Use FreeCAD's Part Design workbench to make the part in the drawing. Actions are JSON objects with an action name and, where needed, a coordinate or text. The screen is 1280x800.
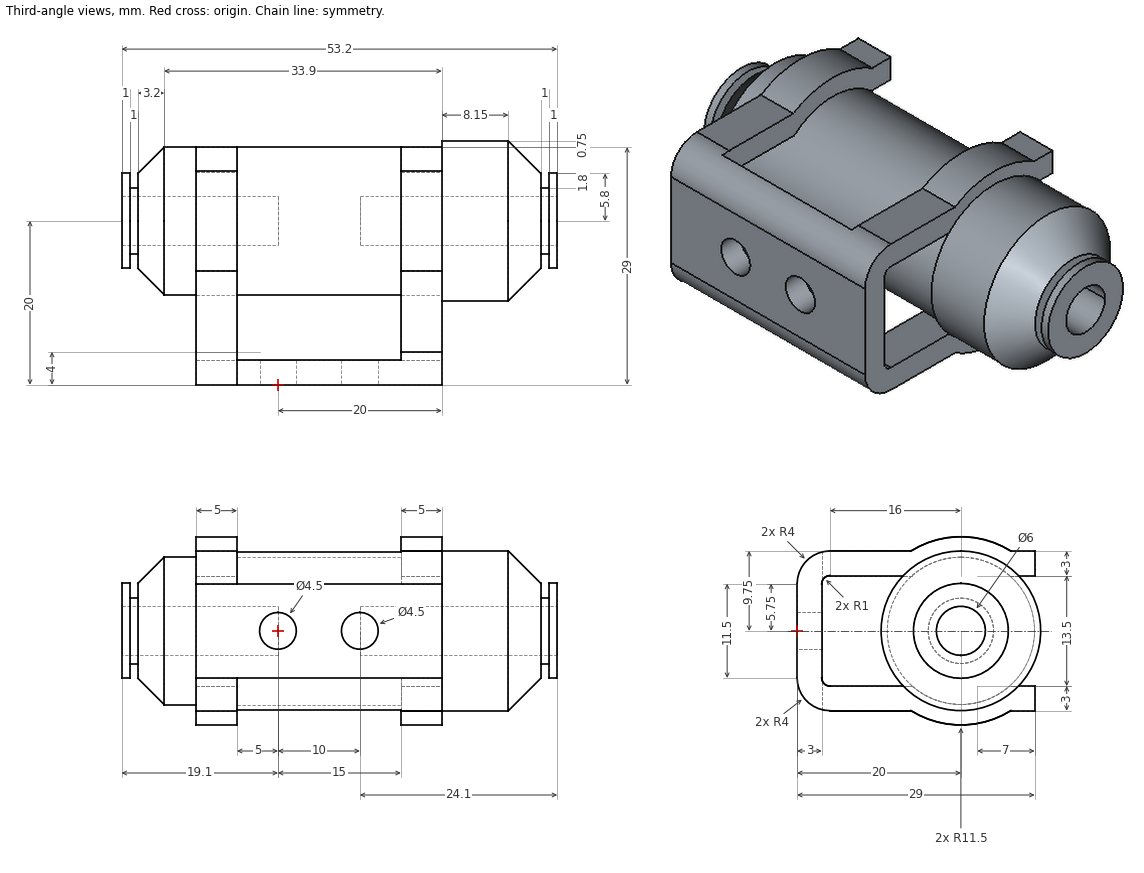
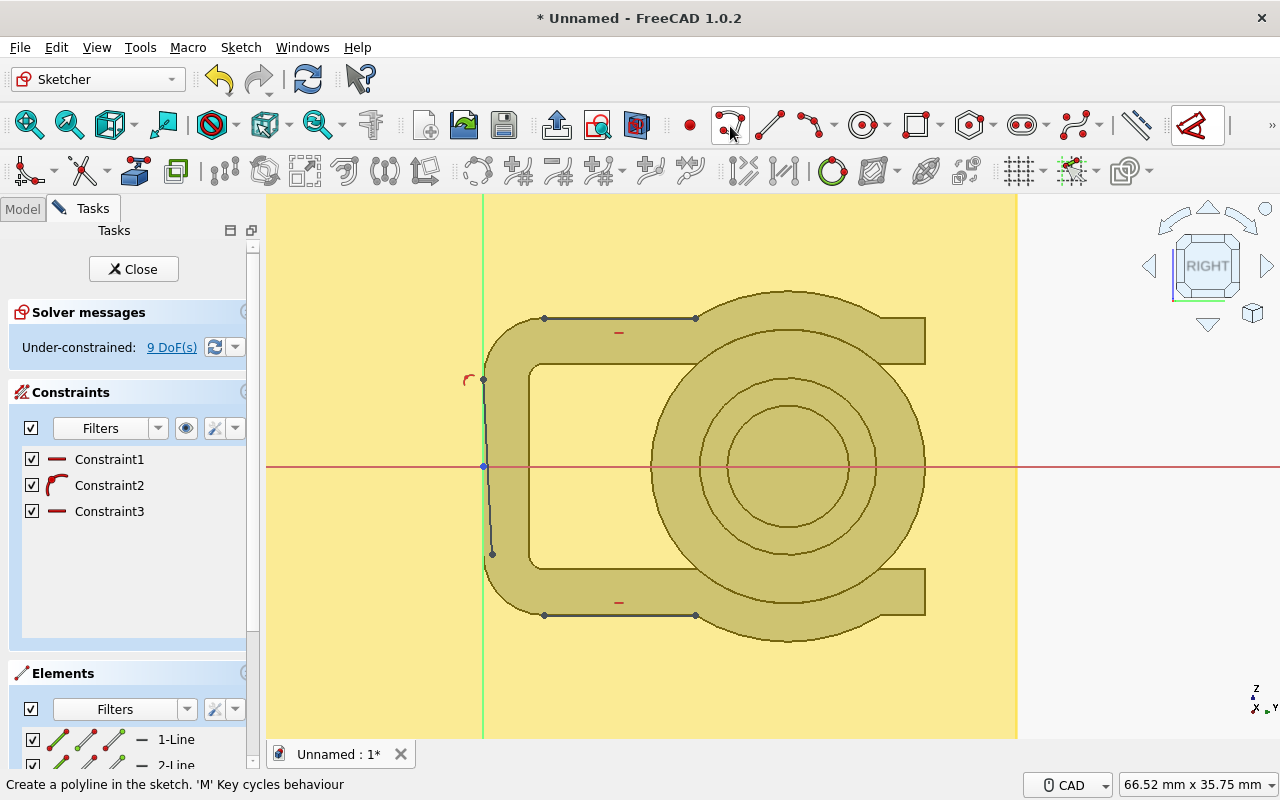
{"action": "left_click", "coordinate": [881, 615]}
{"action": "left_click", "coordinate": [925, 615]}
{"action": "left_click", "coordinate": [925, 569]}
{"action": "left_click", "coordinate": [819, 569]}
{"action": "left_click", "coordinate": [819, 364]}
{"action": "left_click", "coordinate": [925, 364]}
{"action": "left_click", "coordinate": [925, 318]}
{"action": "left_click", "coordinate": [881, 318]}
{"action": "right_click", "coordinate": [881, 318]}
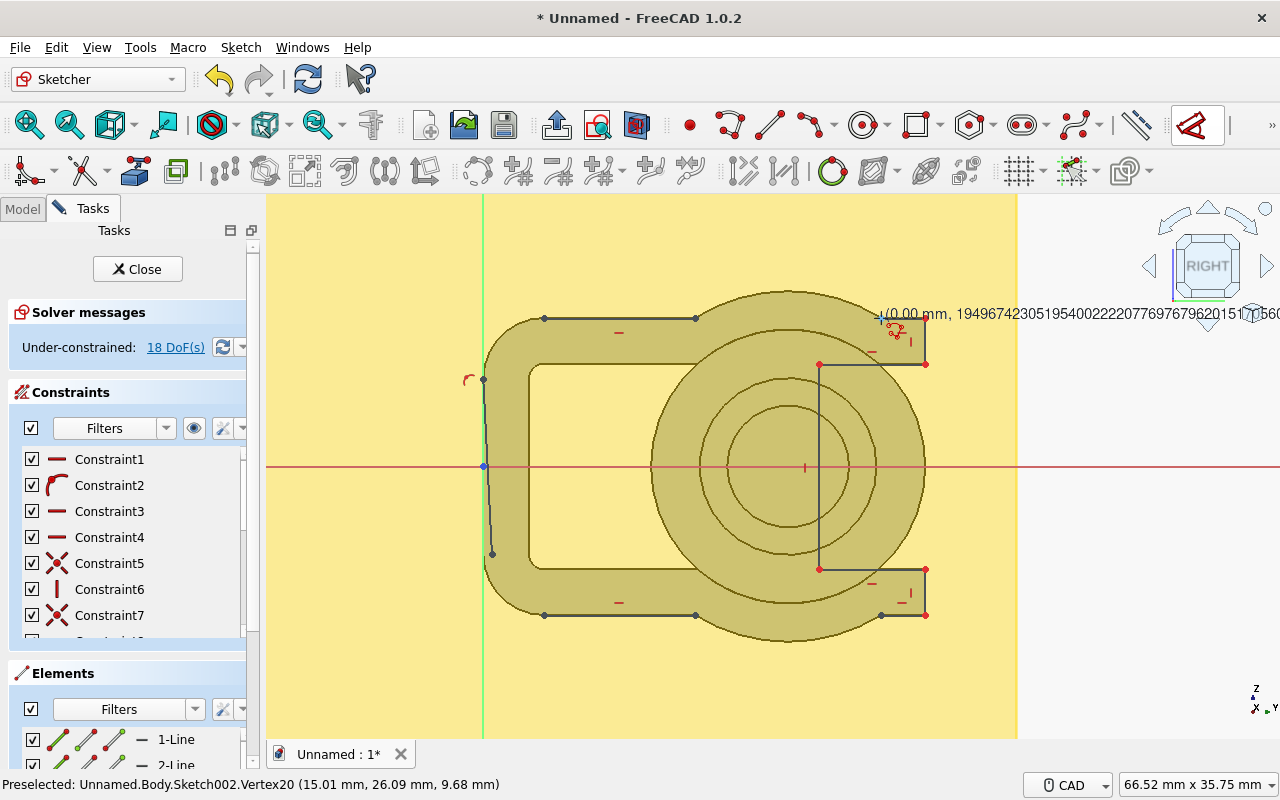
{"action": "left_click", "coordinate": [810, 126]}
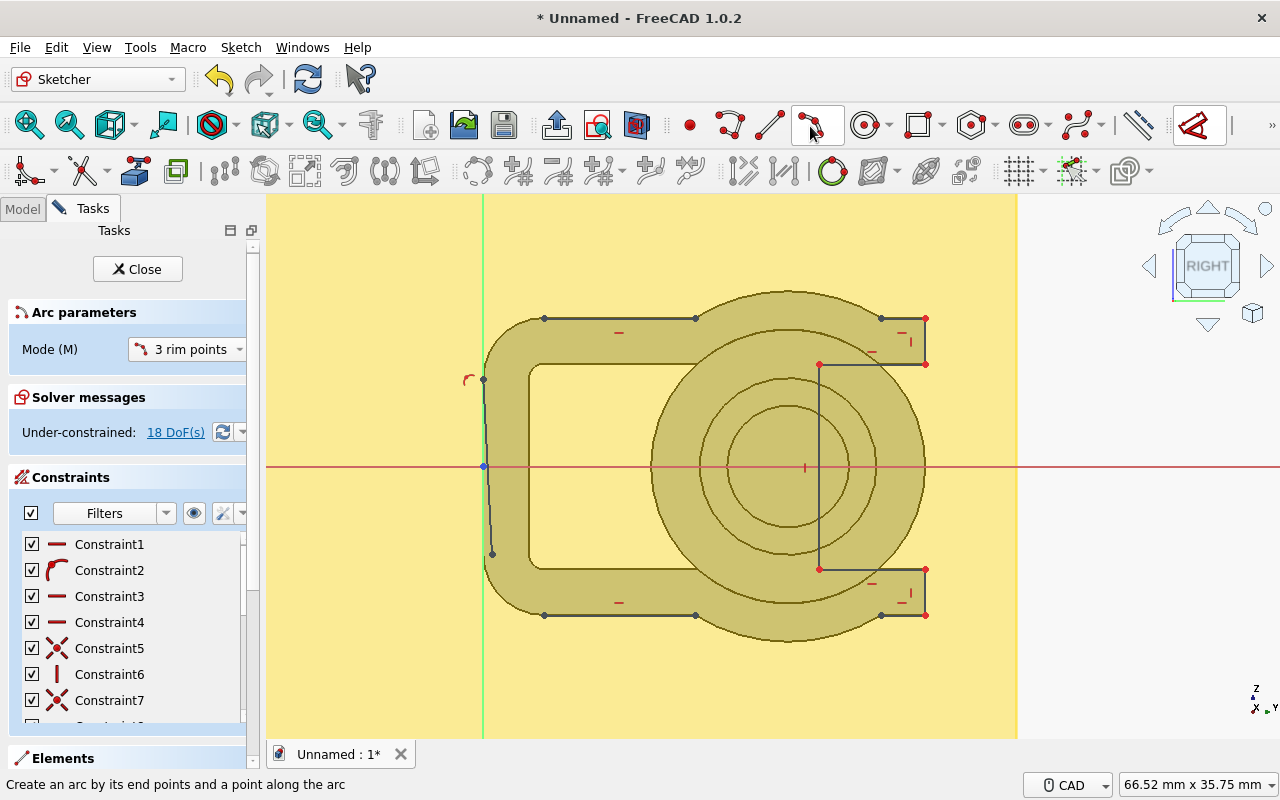
{"action": "left_click", "coordinate": [544, 319]}
{"action": "left_click", "coordinate": [483, 380]}
{"action": "left_click", "coordinate": [501, 336]}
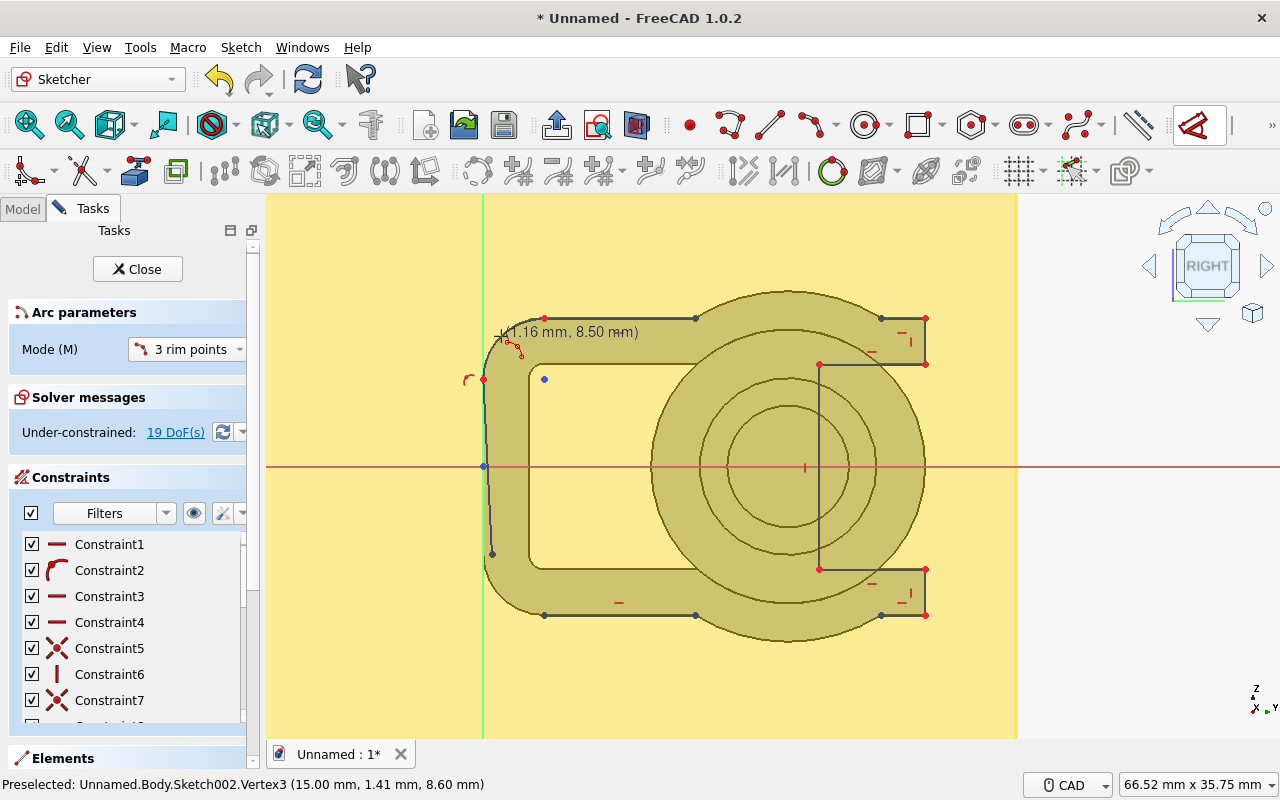
{"action": "left_click", "coordinate": [492, 555]}
{"action": "left_click", "coordinate": [544, 616]}
{"action": "left_click", "coordinate": [501, 597]}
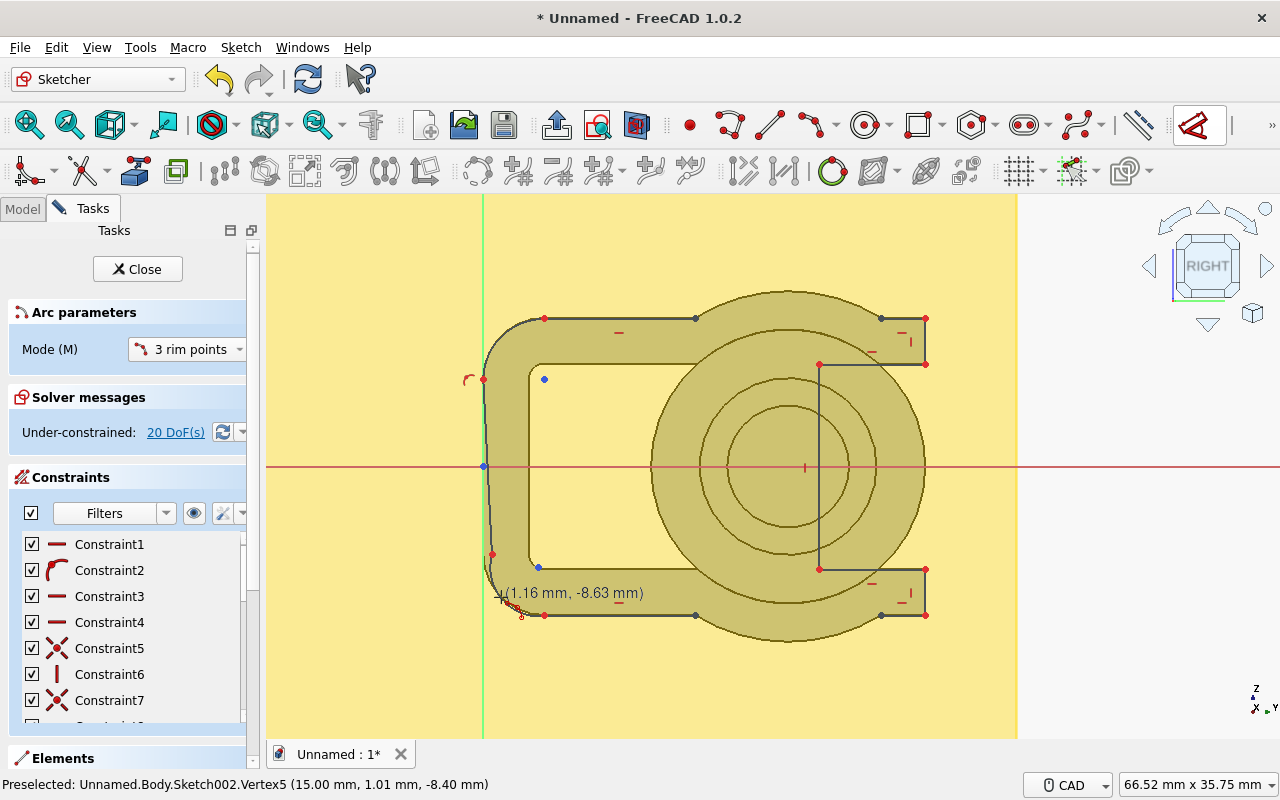
{"action": "left_click", "coordinate": [695, 616]}
{"action": "left_click", "coordinate": [881, 616]}
{"action": "left_click", "coordinate": [788, 642]}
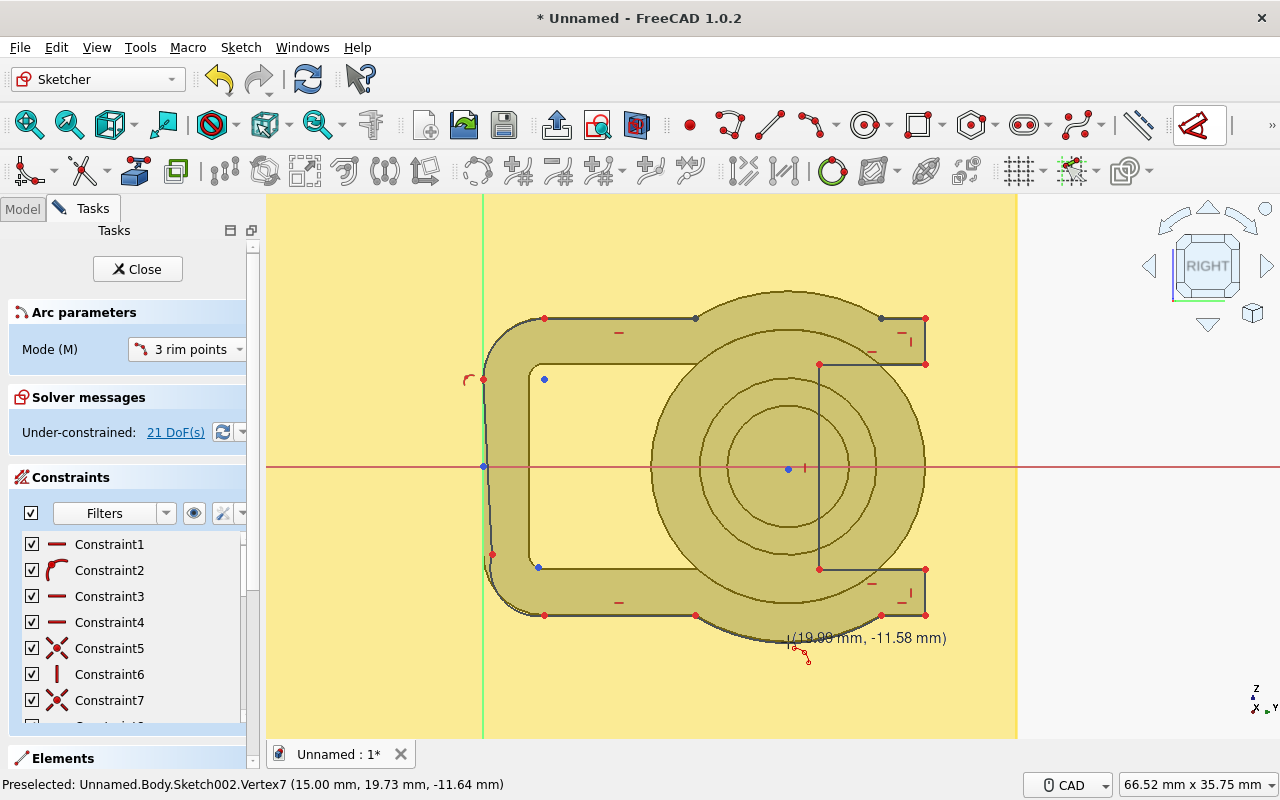
{"action": "left_click", "coordinate": [881, 319]}
{"action": "left_click", "coordinate": [695, 319]}
{"action": "left_click", "coordinate": [788, 291]}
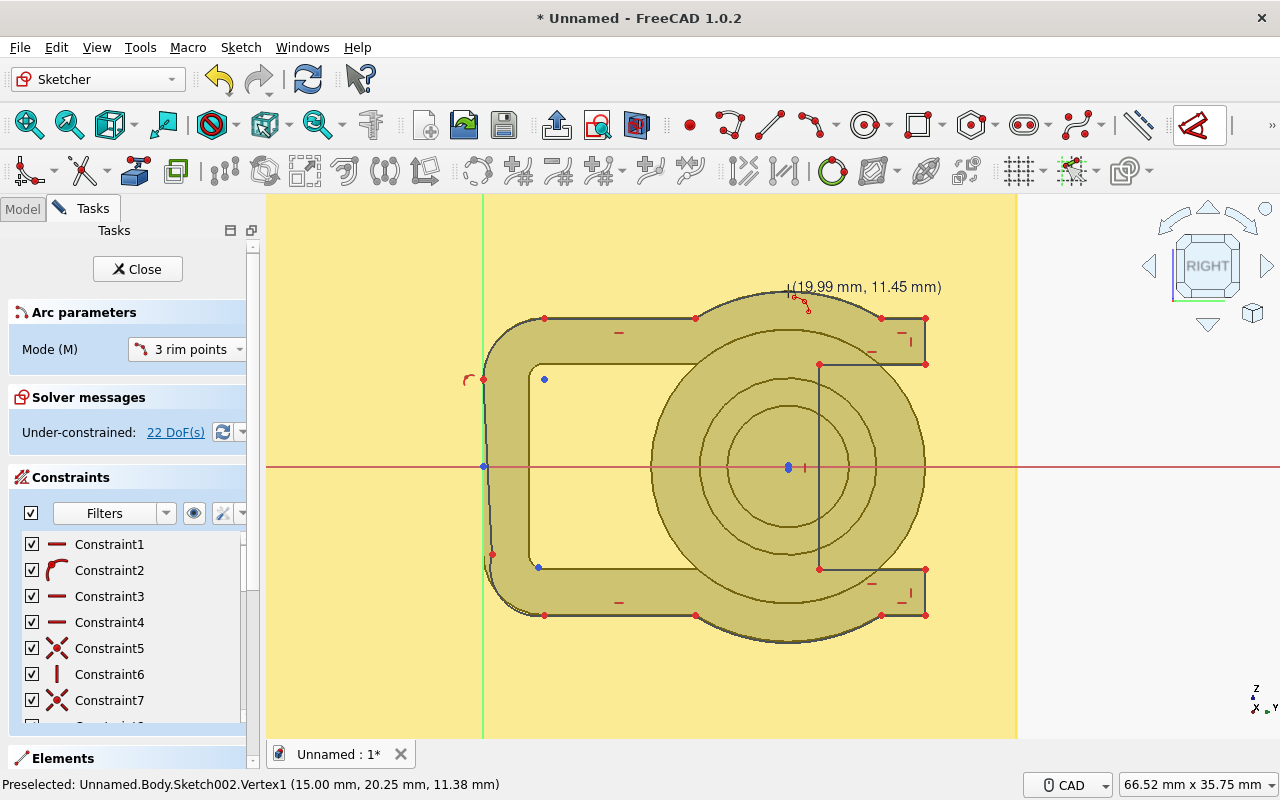
{"action": "left_click", "coordinate": [770, 126]}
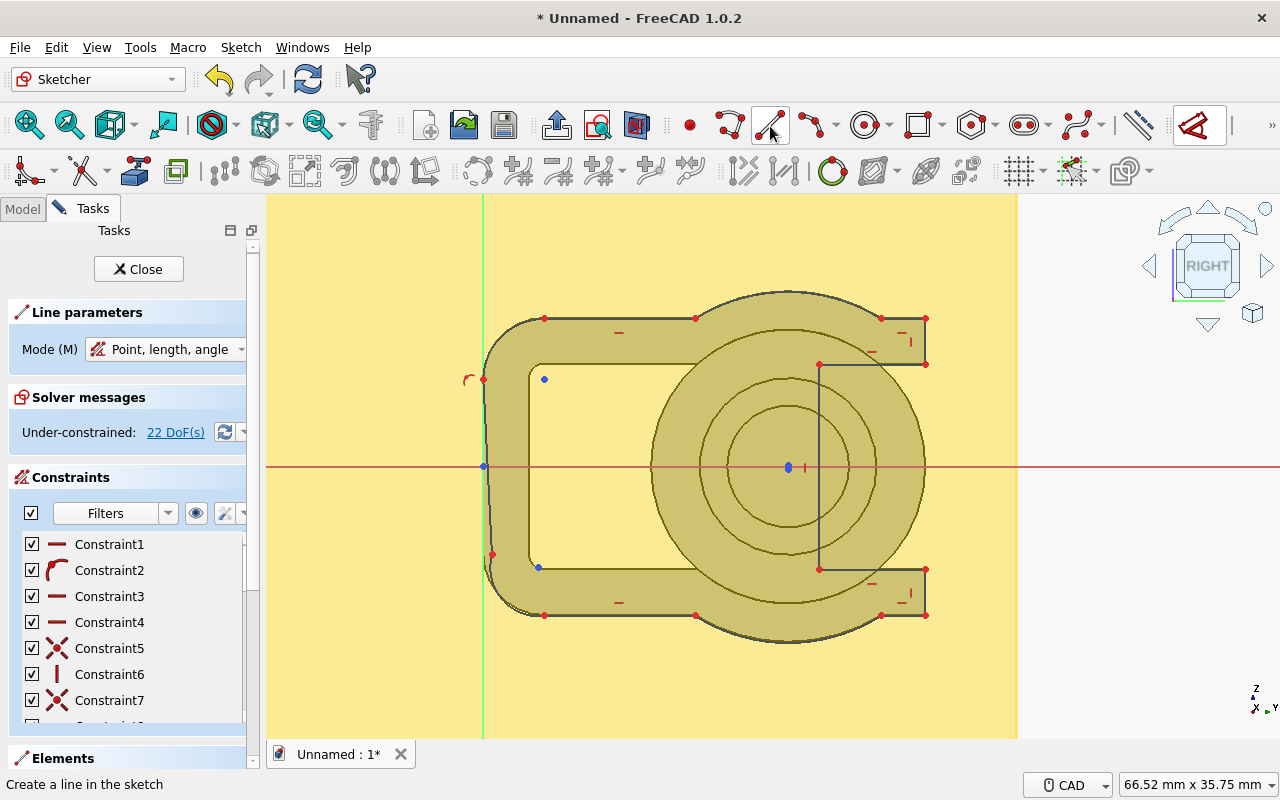
{"action": "left_click", "coordinate": [529, 554]}
{"action": "left_click", "coordinate": [529, 379]}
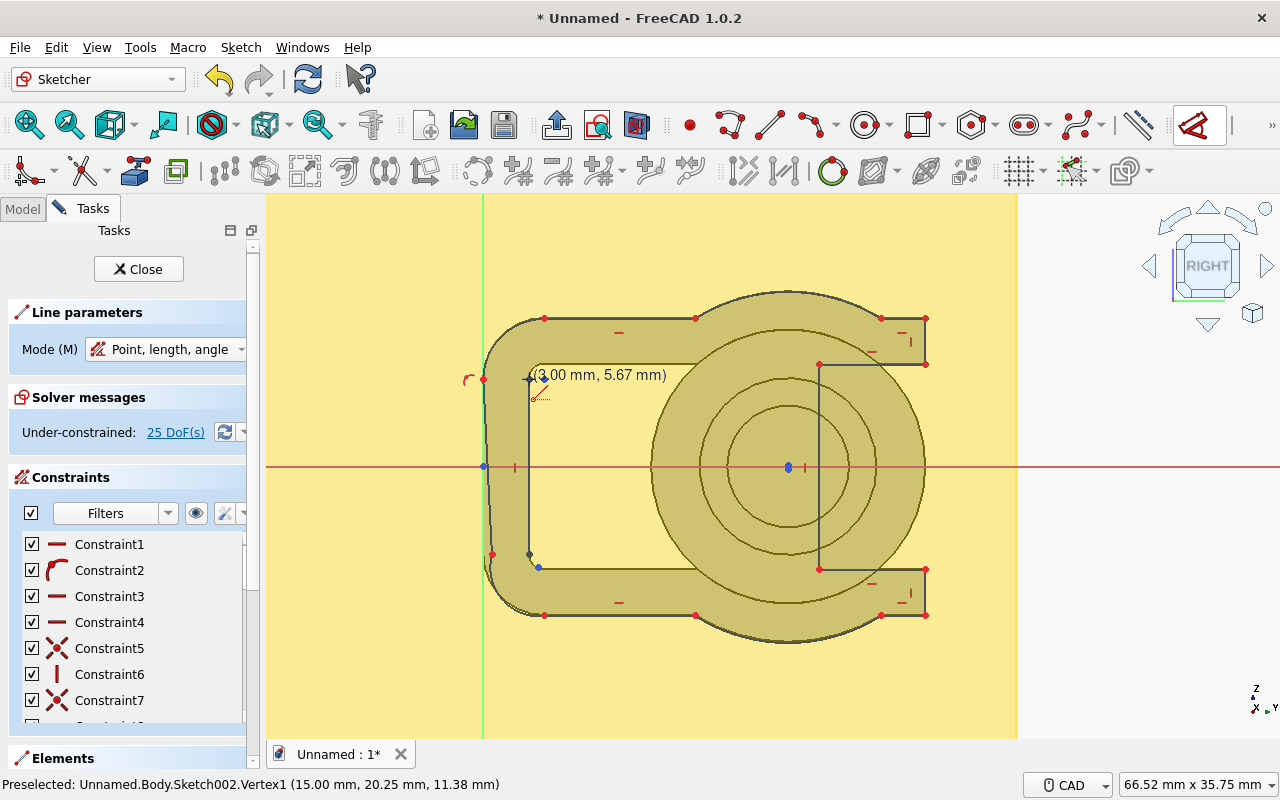
{"action": "left_click", "coordinate": [730, 126]}